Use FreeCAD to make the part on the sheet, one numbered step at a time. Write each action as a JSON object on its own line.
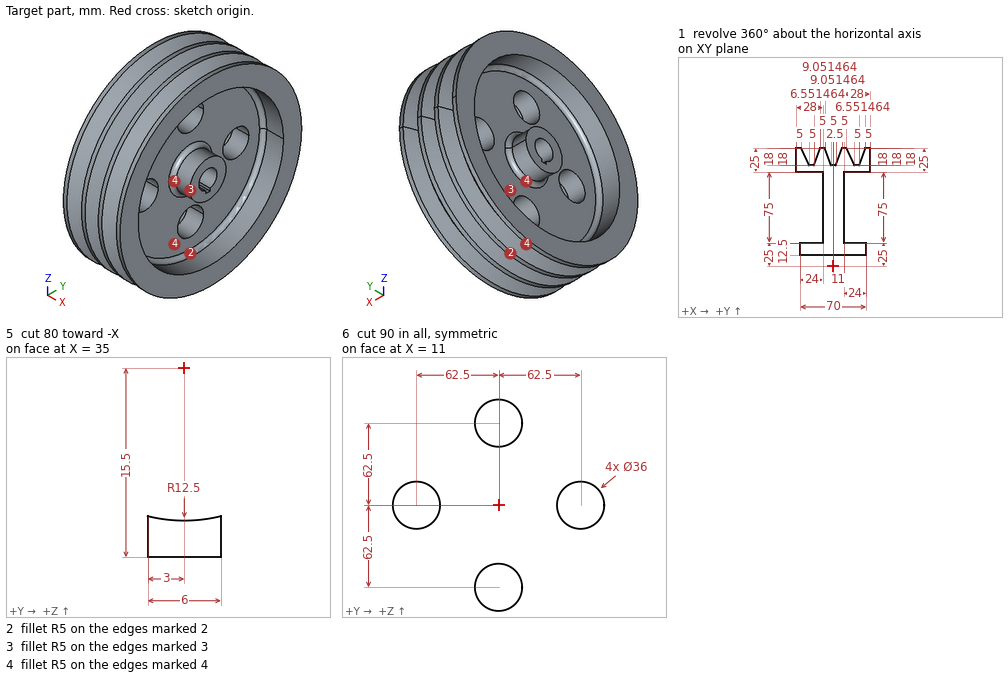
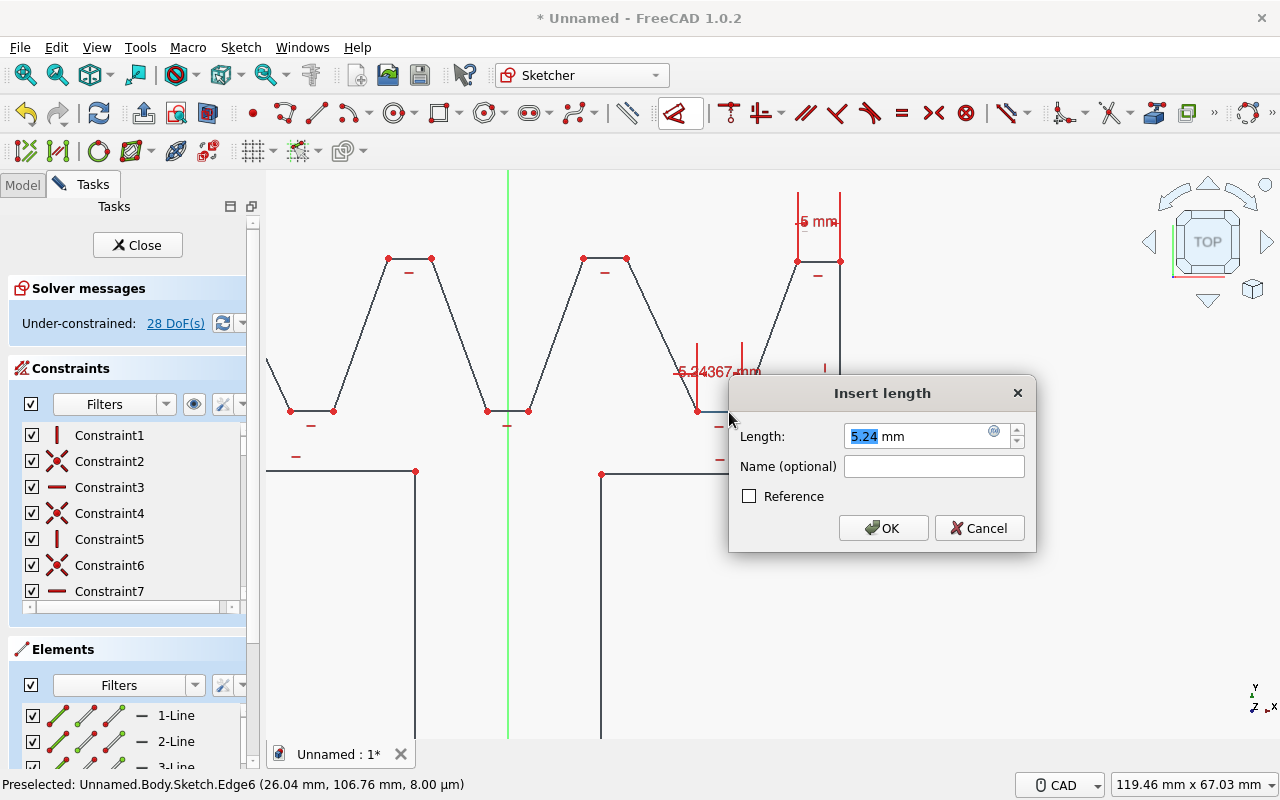
{"action": "type", "text": "5"}
{"action": "key", "text": "Return"}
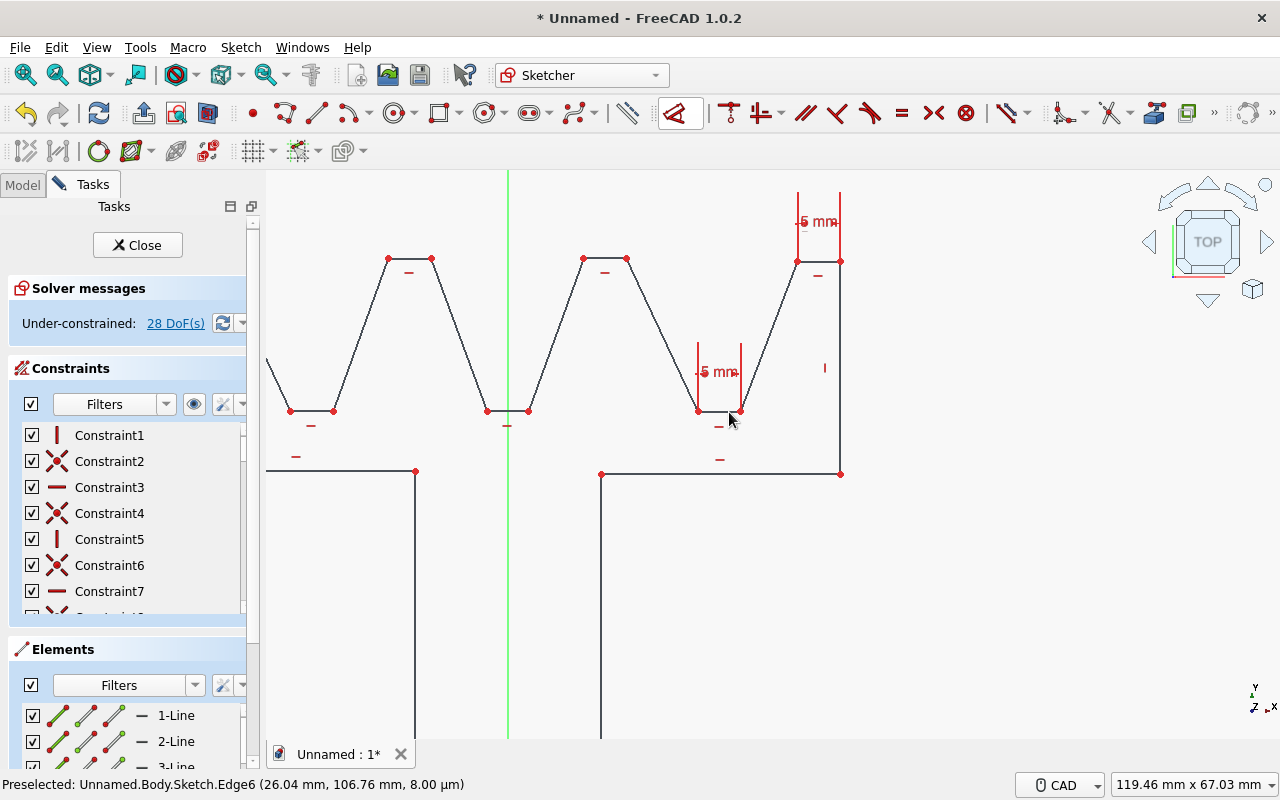
{"action": "left_click", "coordinate": [614, 258]}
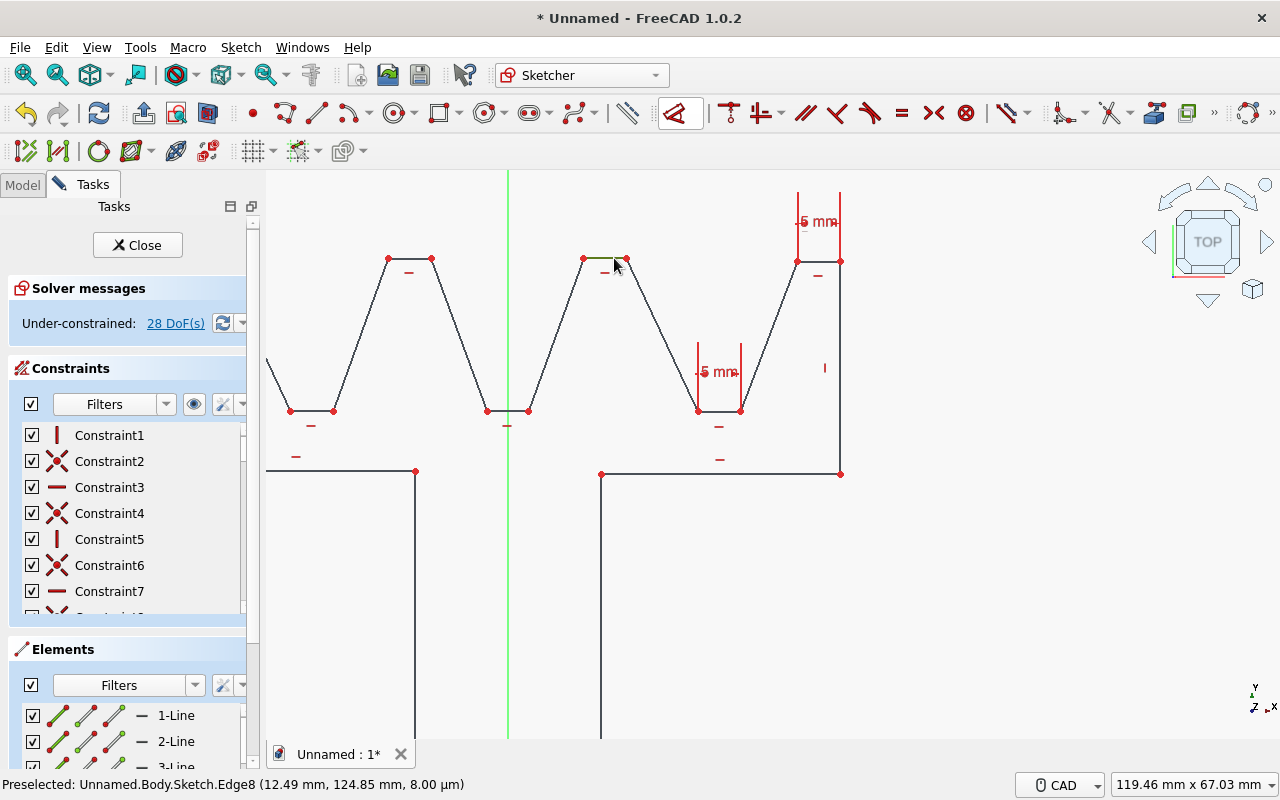
{"action": "key", "text": "l"}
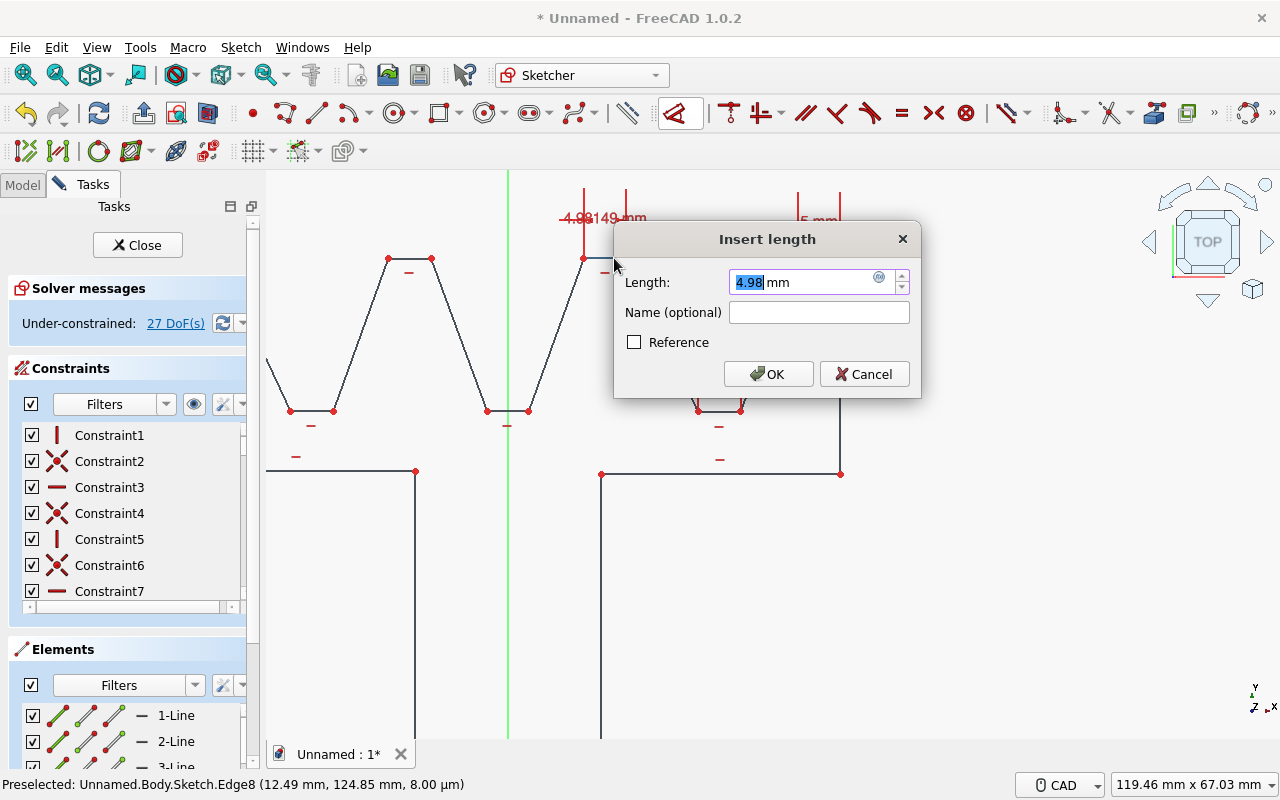
{"action": "type", "text": "5"}
{"action": "key", "text": "Return"}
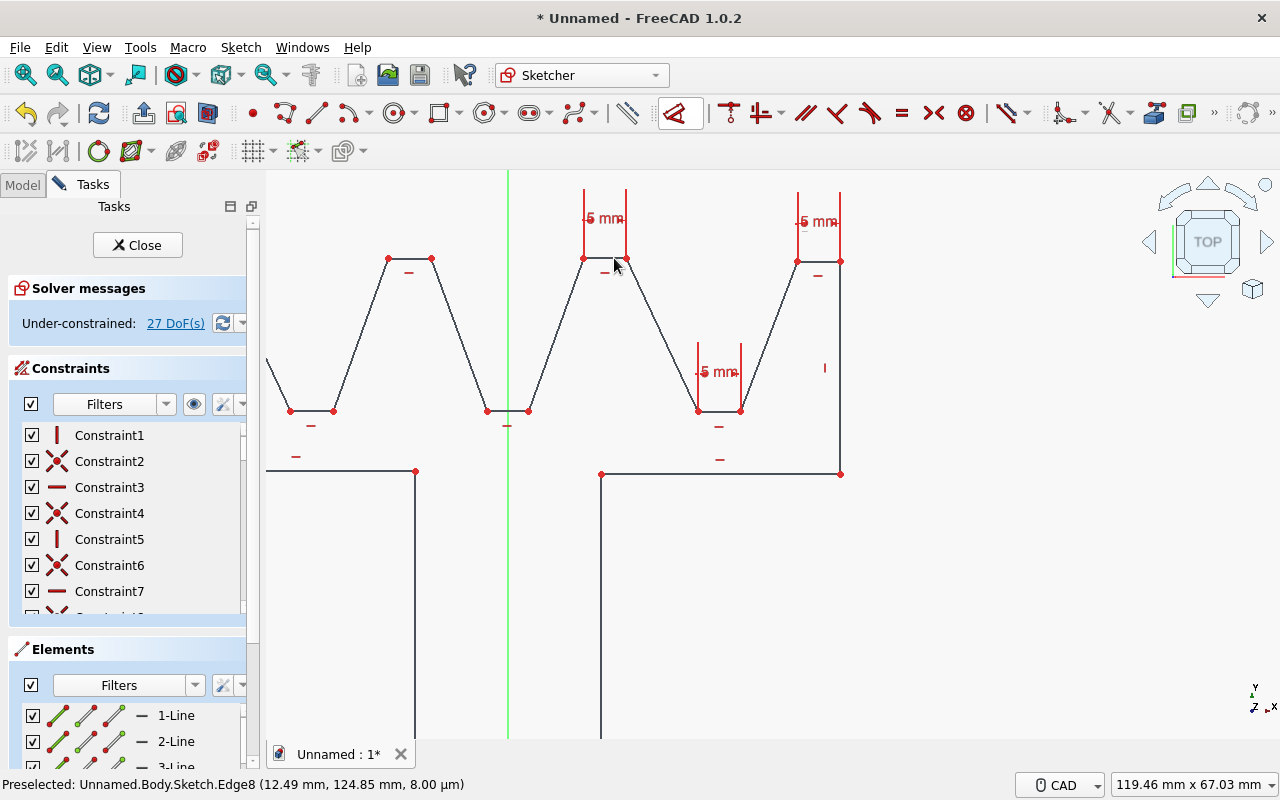
{"action": "left_click", "coordinate": [508, 411]}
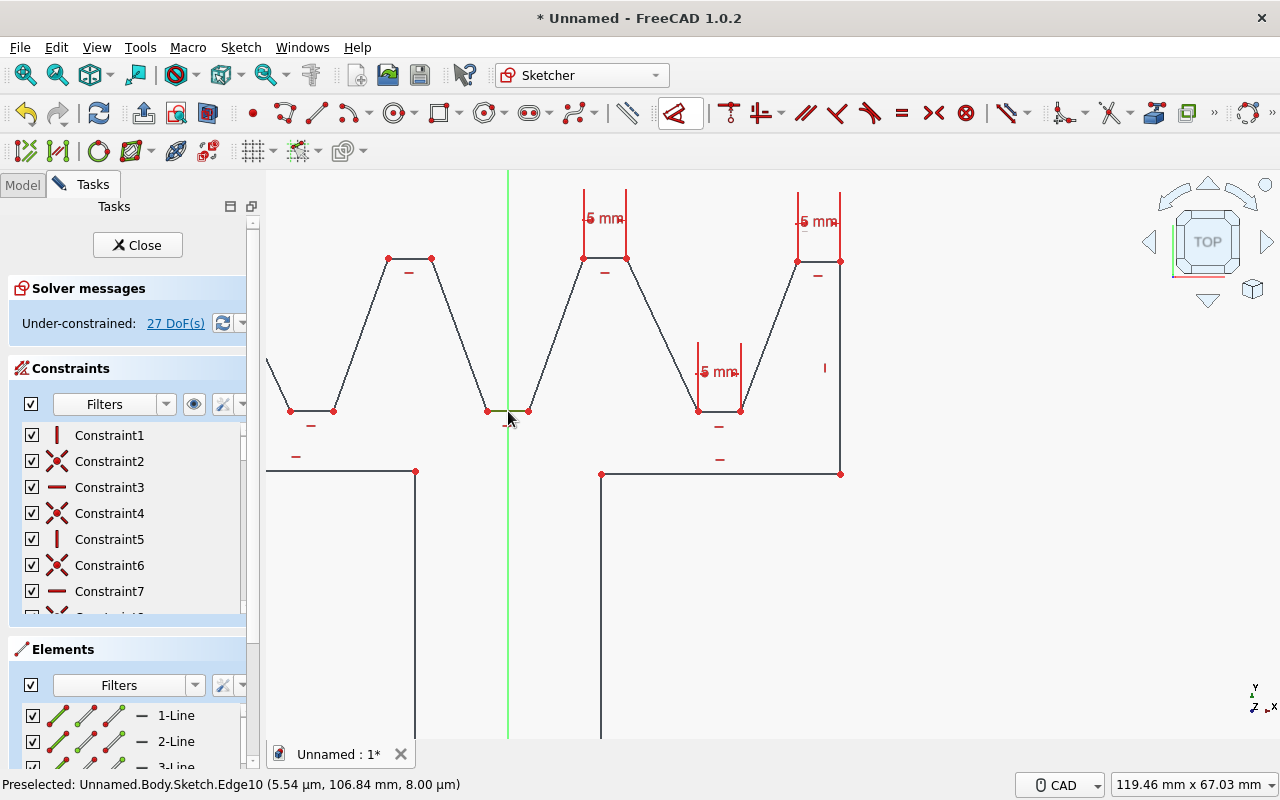
{"action": "left_click", "coordinate": [698, 114]}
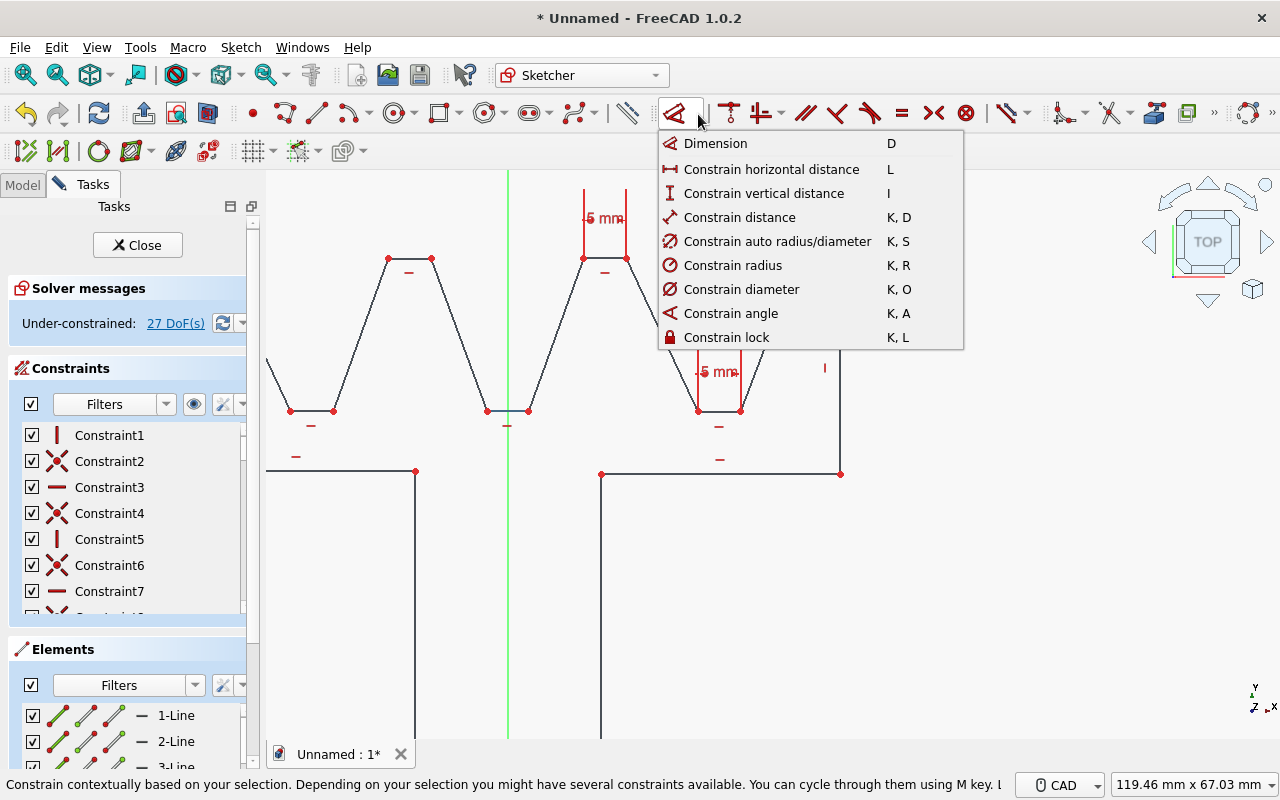
{"action": "left_click", "coordinate": [811, 169]}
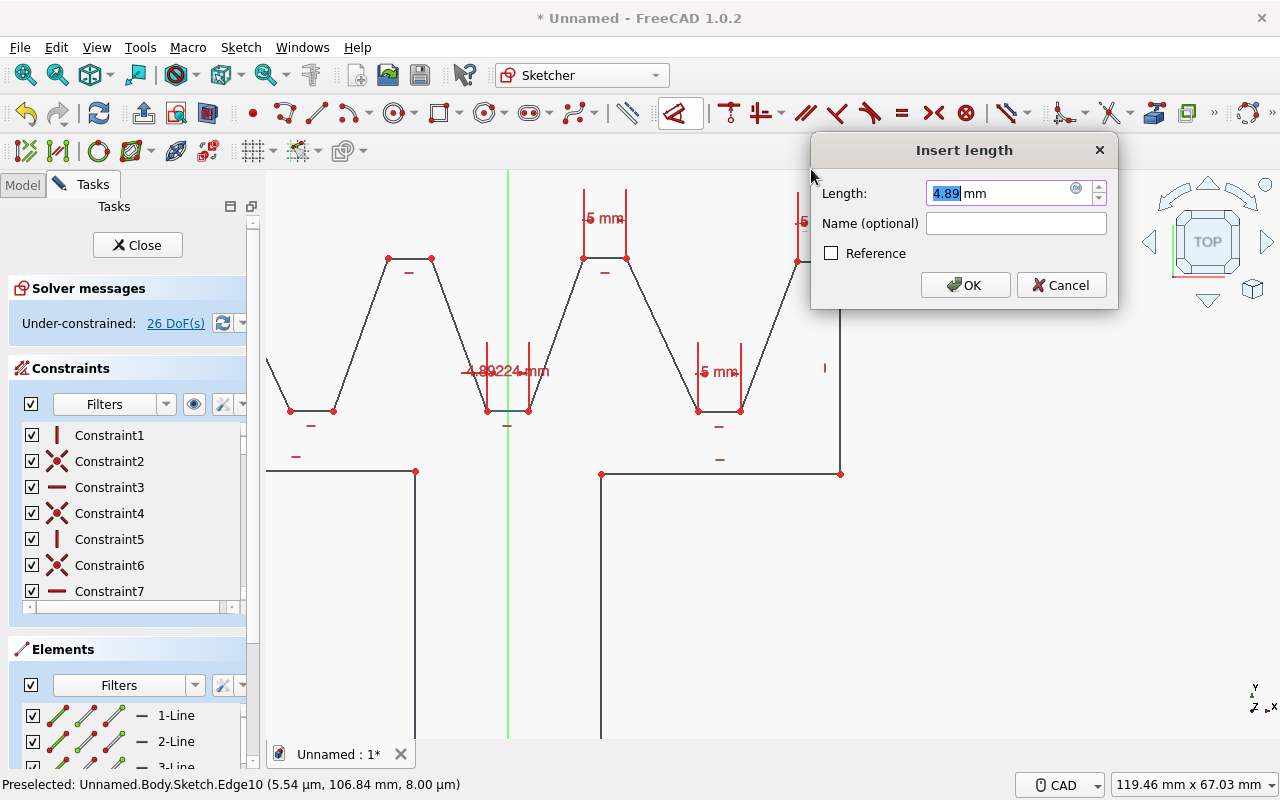
{"action": "type", "text": "5"}
{"action": "key", "text": "Return"}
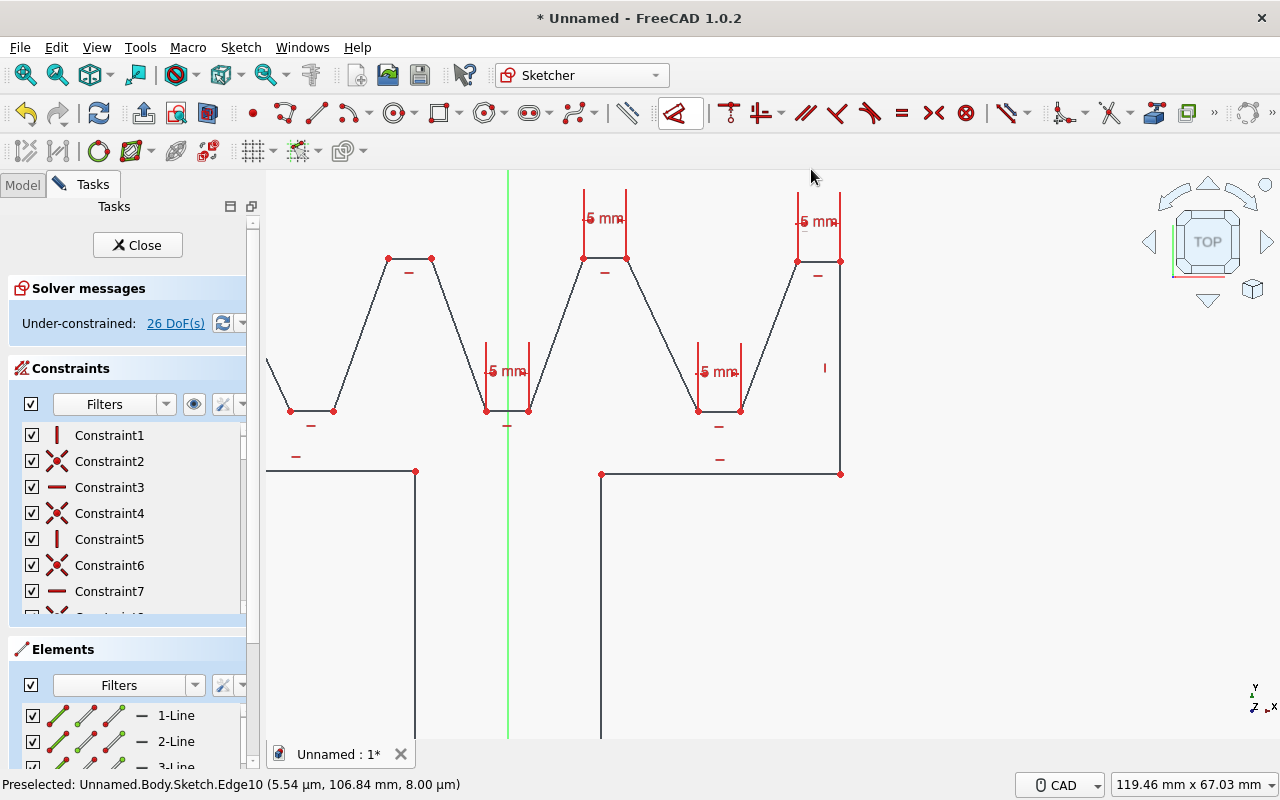
{"action": "left_click", "coordinate": [418, 259]}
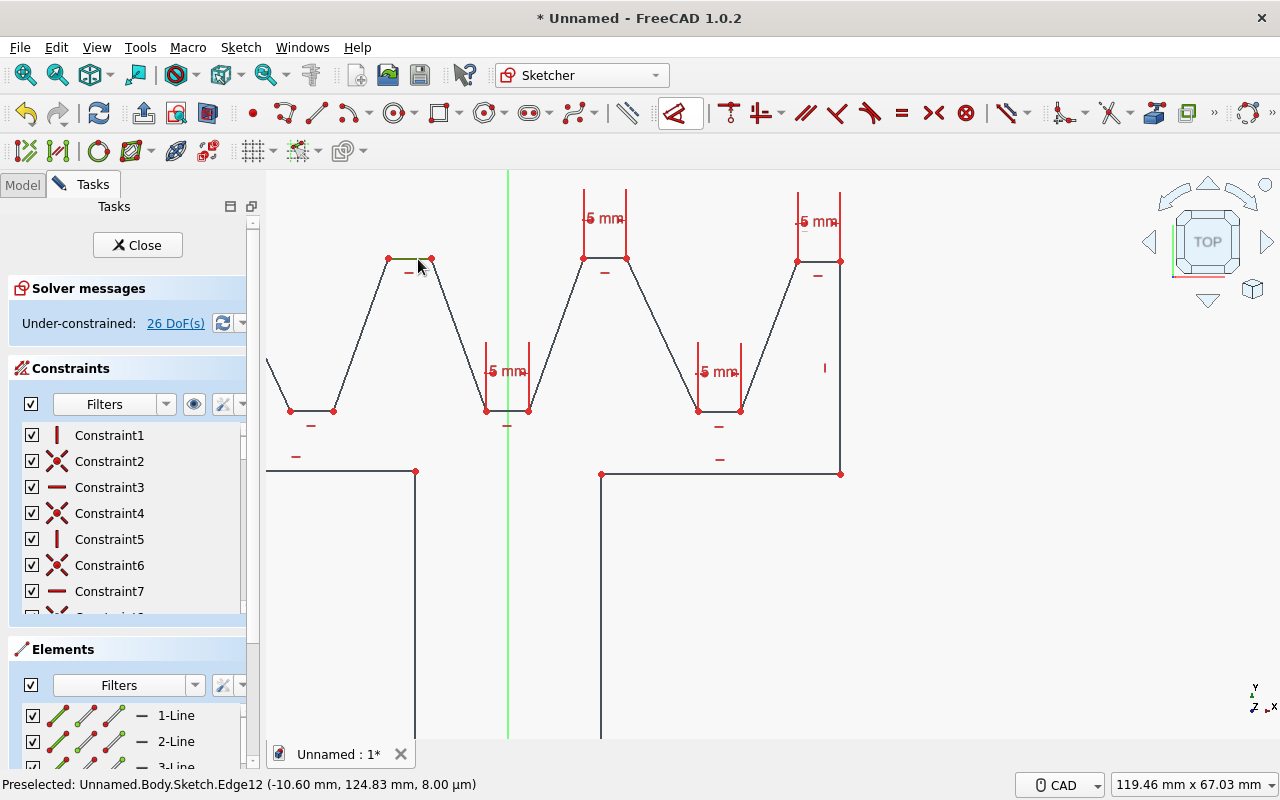
{"action": "left_click", "coordinate": [698, 114]}